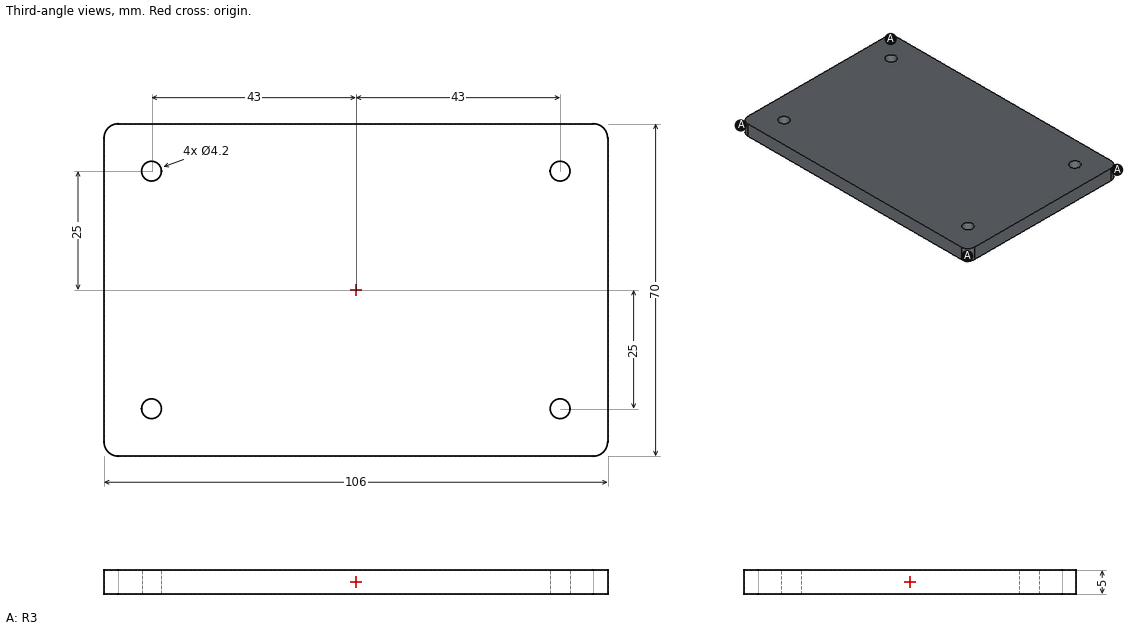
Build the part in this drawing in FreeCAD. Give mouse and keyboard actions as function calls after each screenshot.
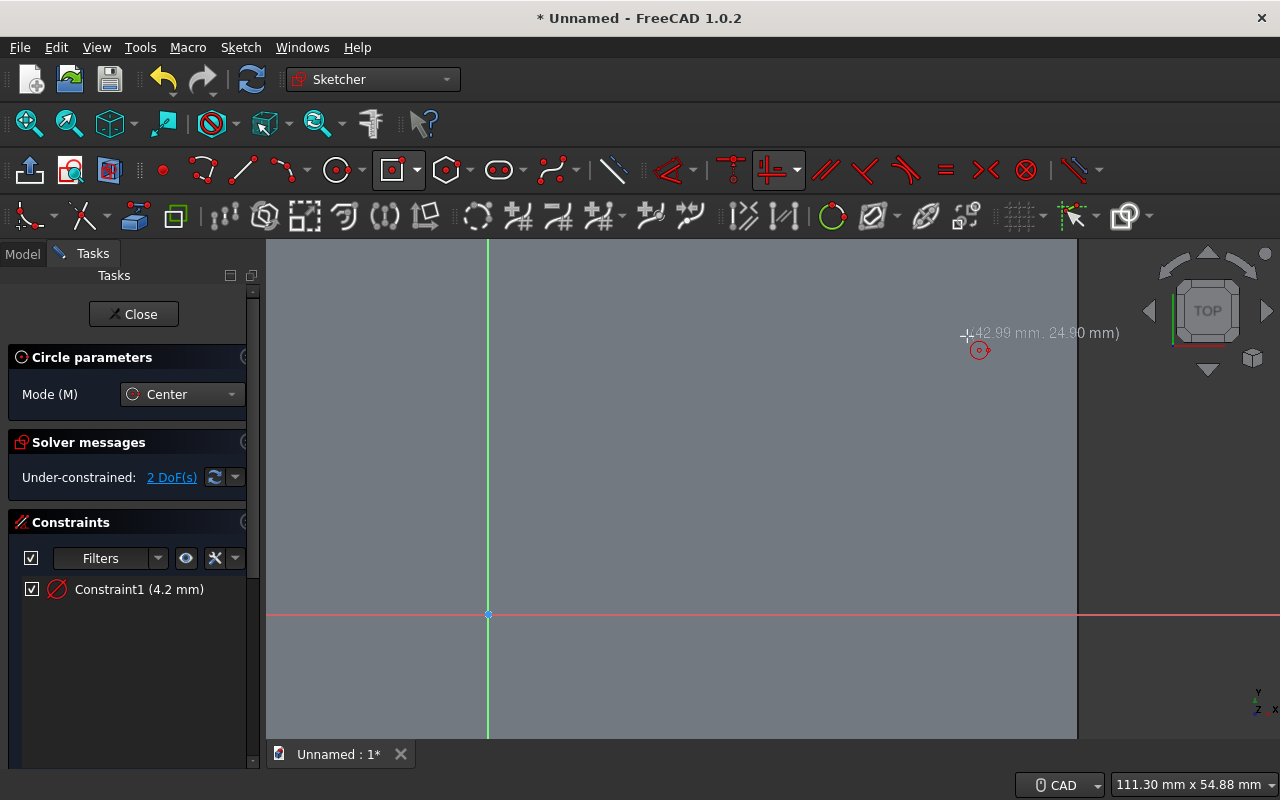
click(967, 337)
move(983, 320)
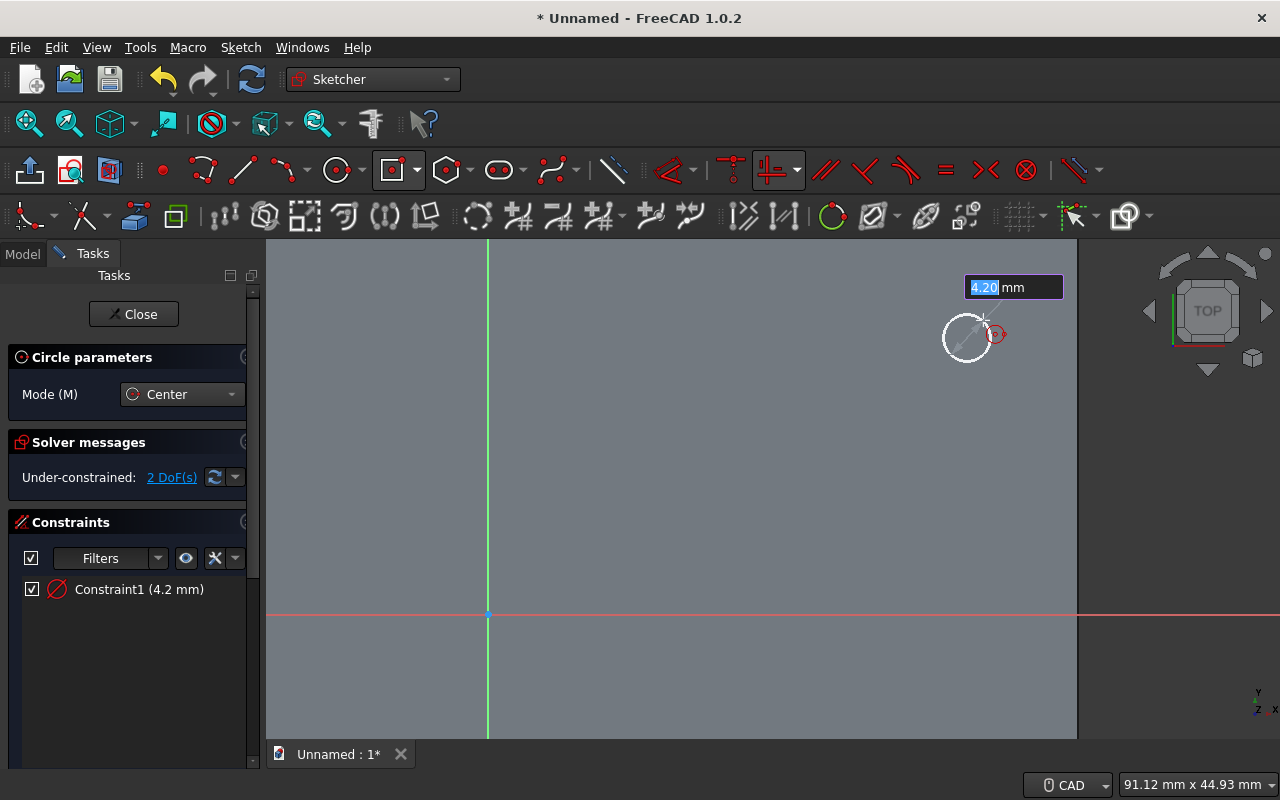
text(4.2)
key(Return)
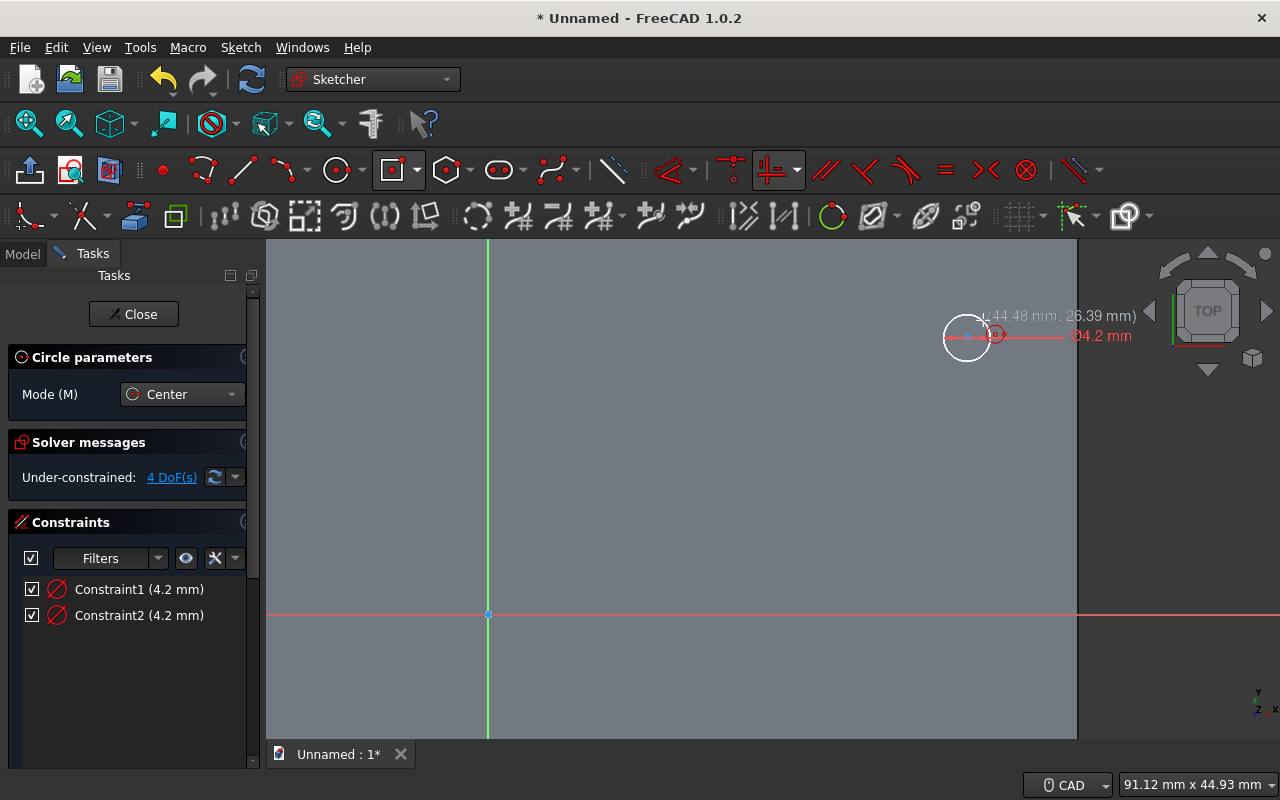
scroll(968, 336, down, 3)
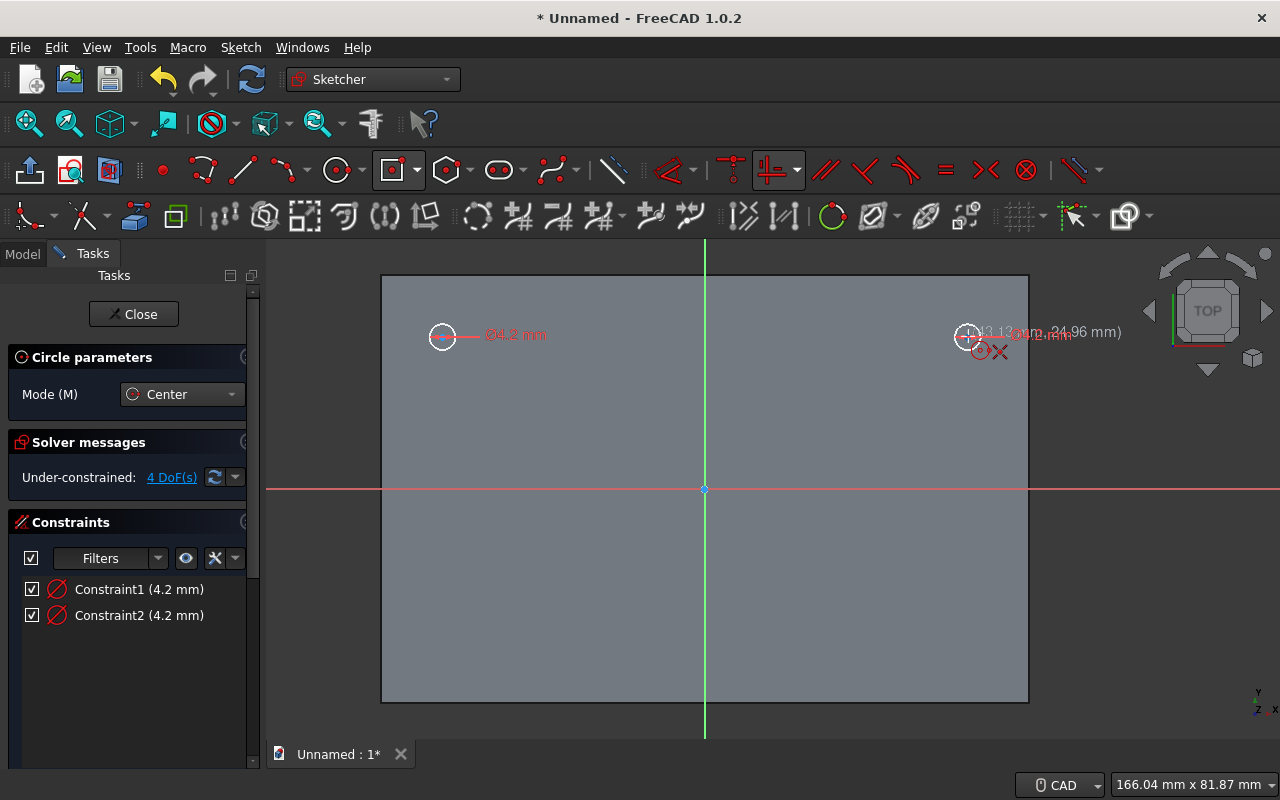
scroll(968, 642, up, 3)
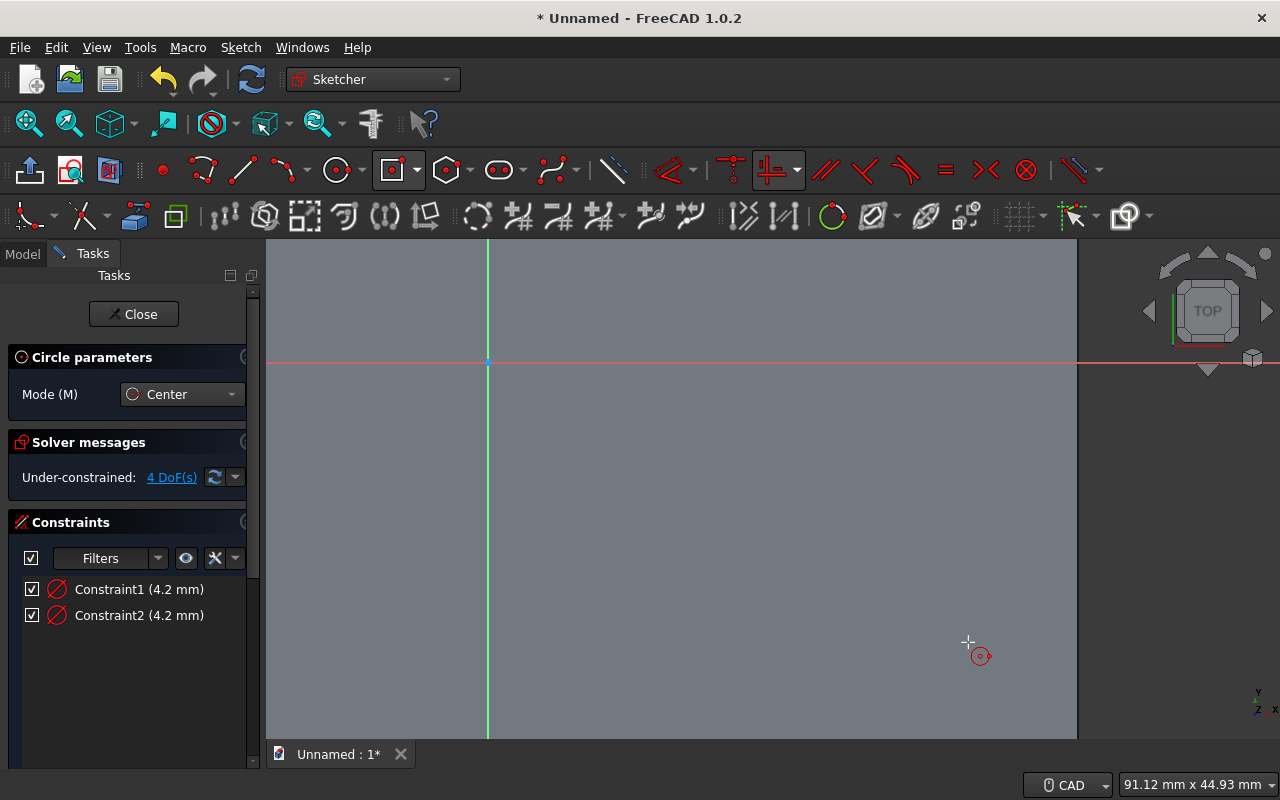
click(967, 641)
move(983, 624)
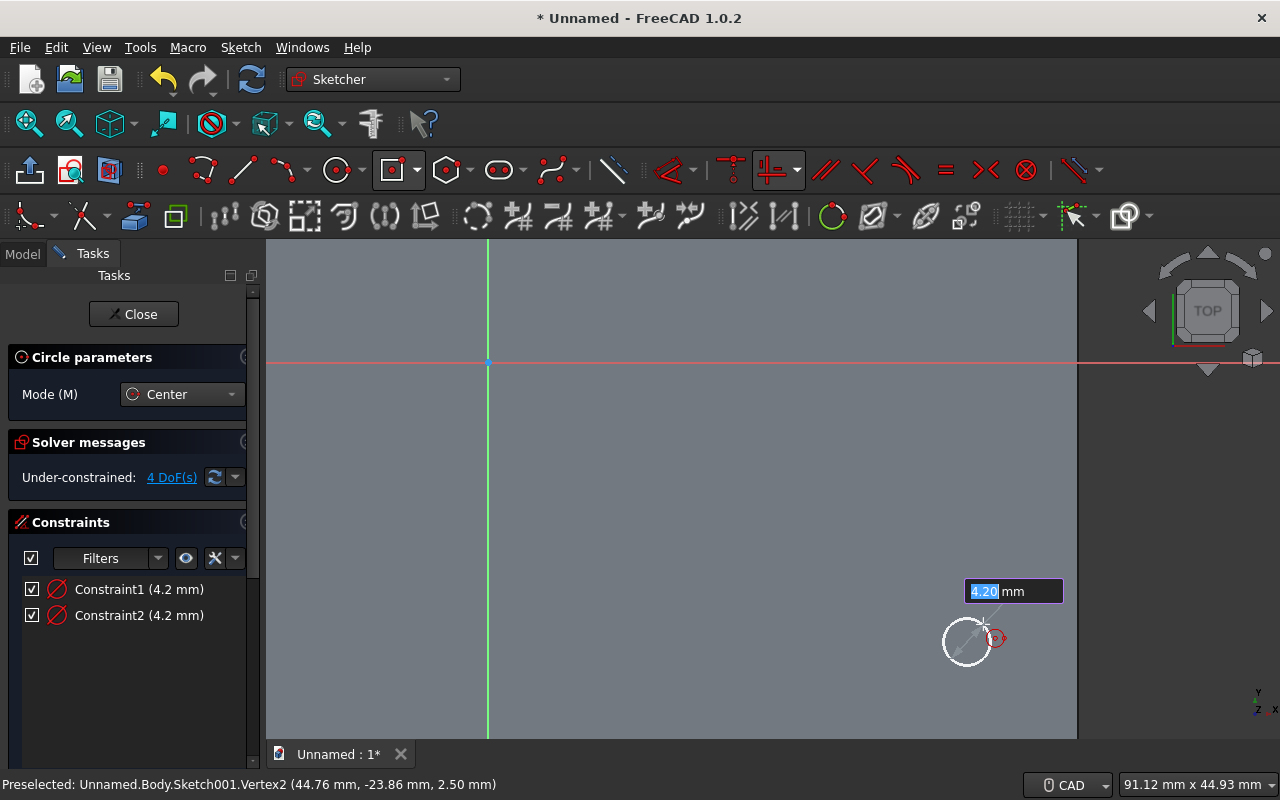
text(4.2)
key(Return)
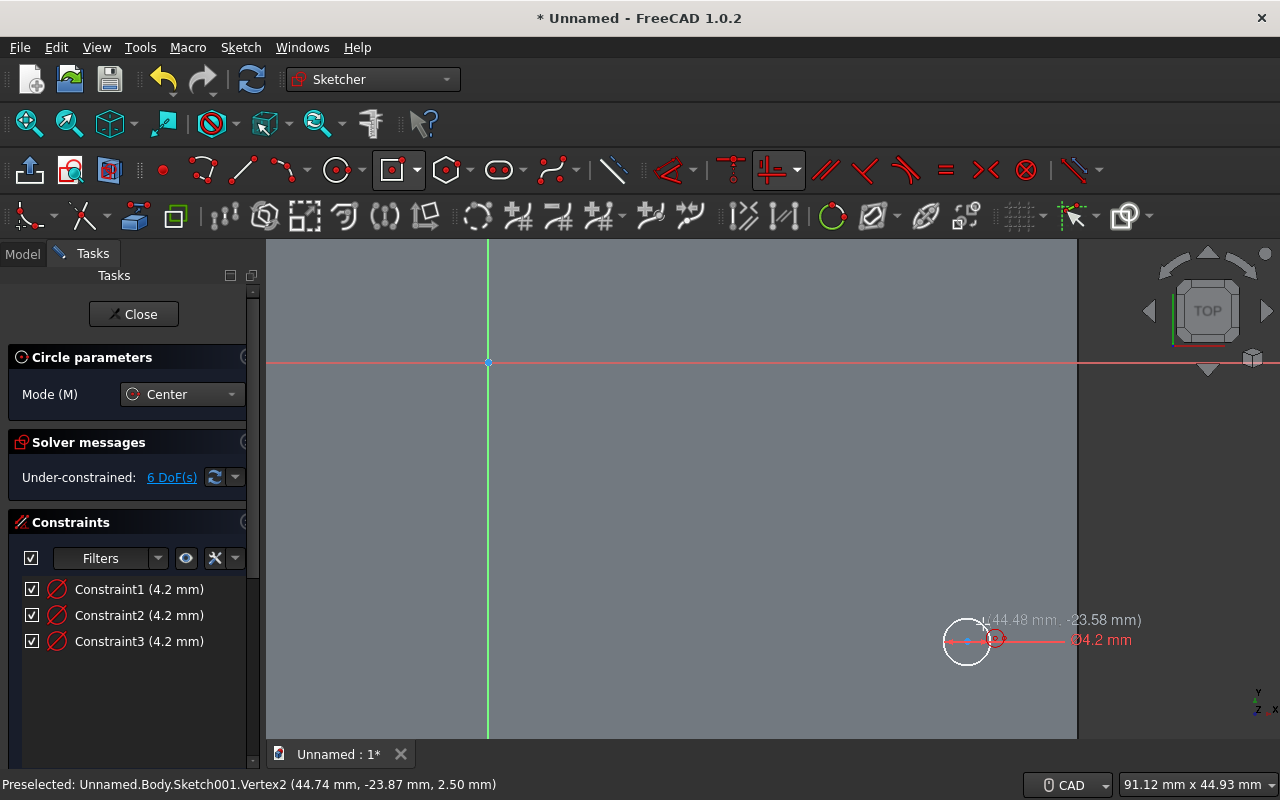
scroll(968, 643, down, 3)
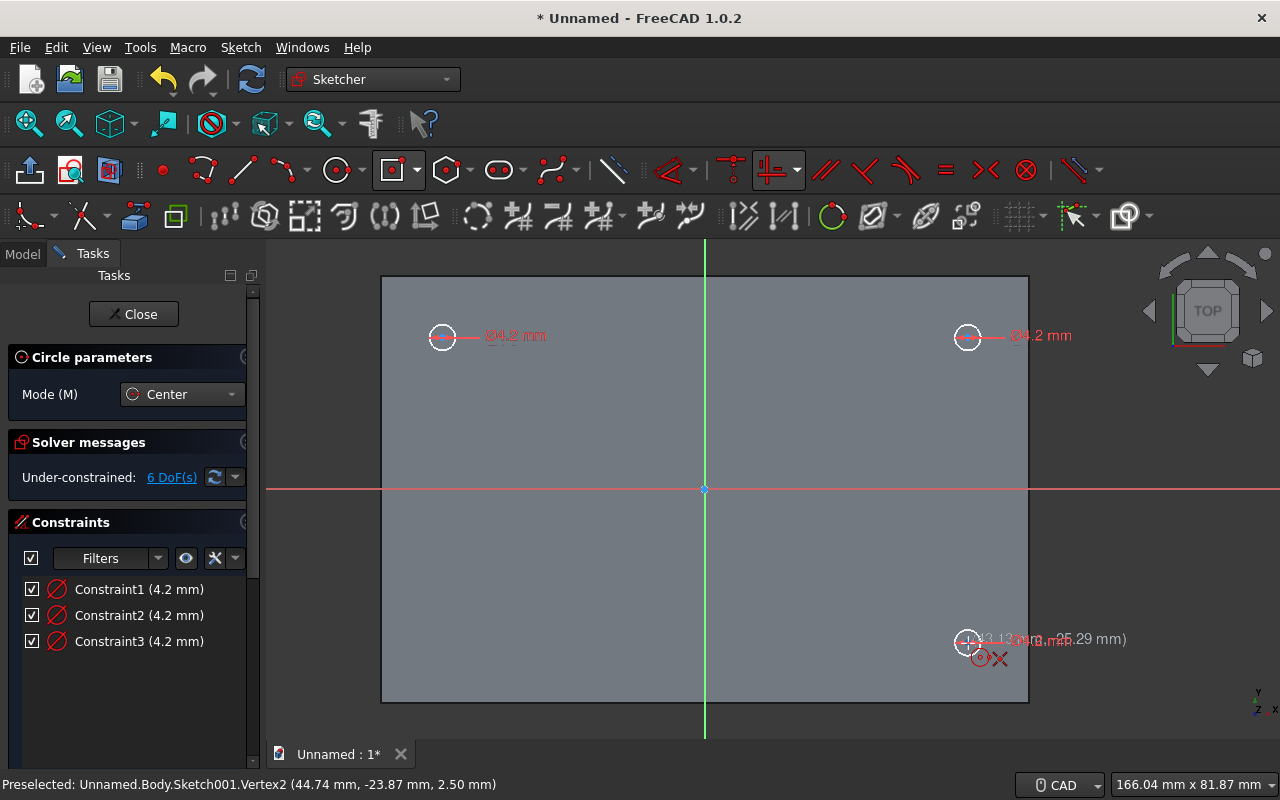
scroll(442, 642, up, 3)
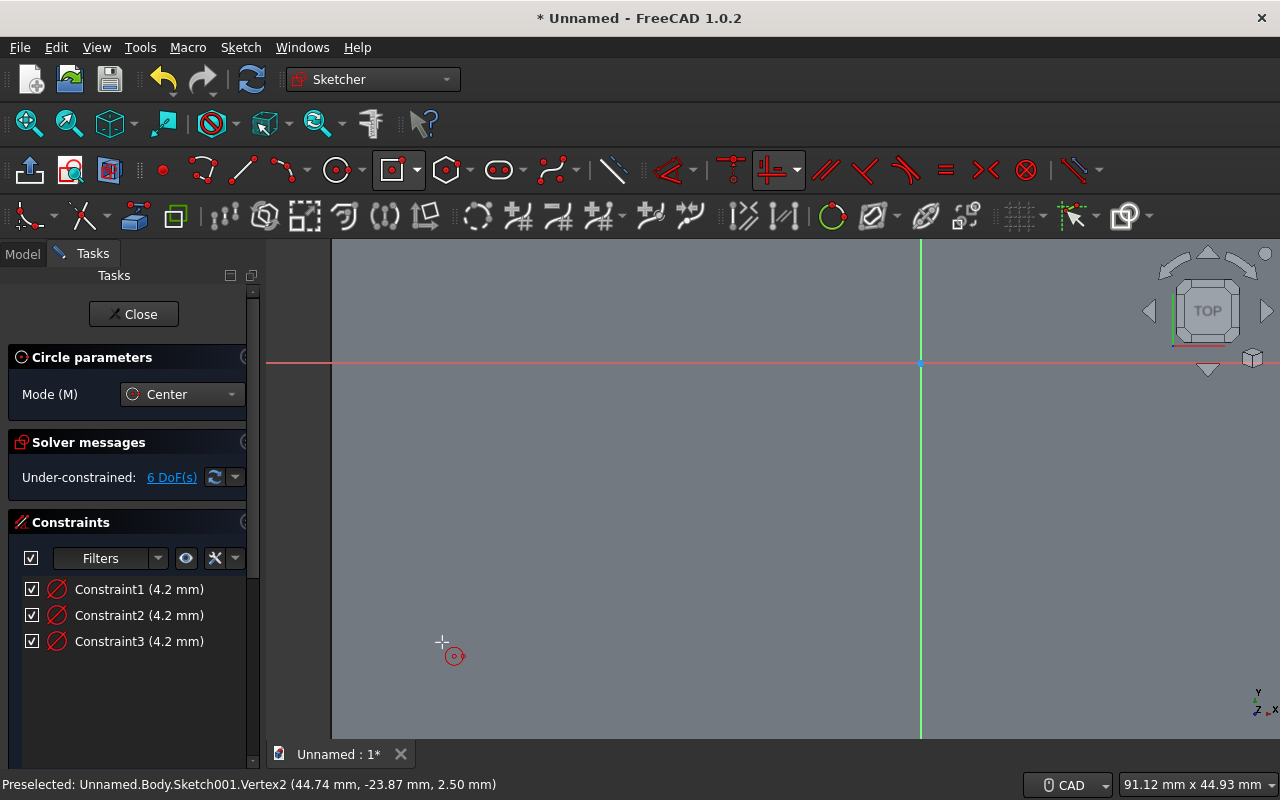
click(442, 642)
move(459, 625)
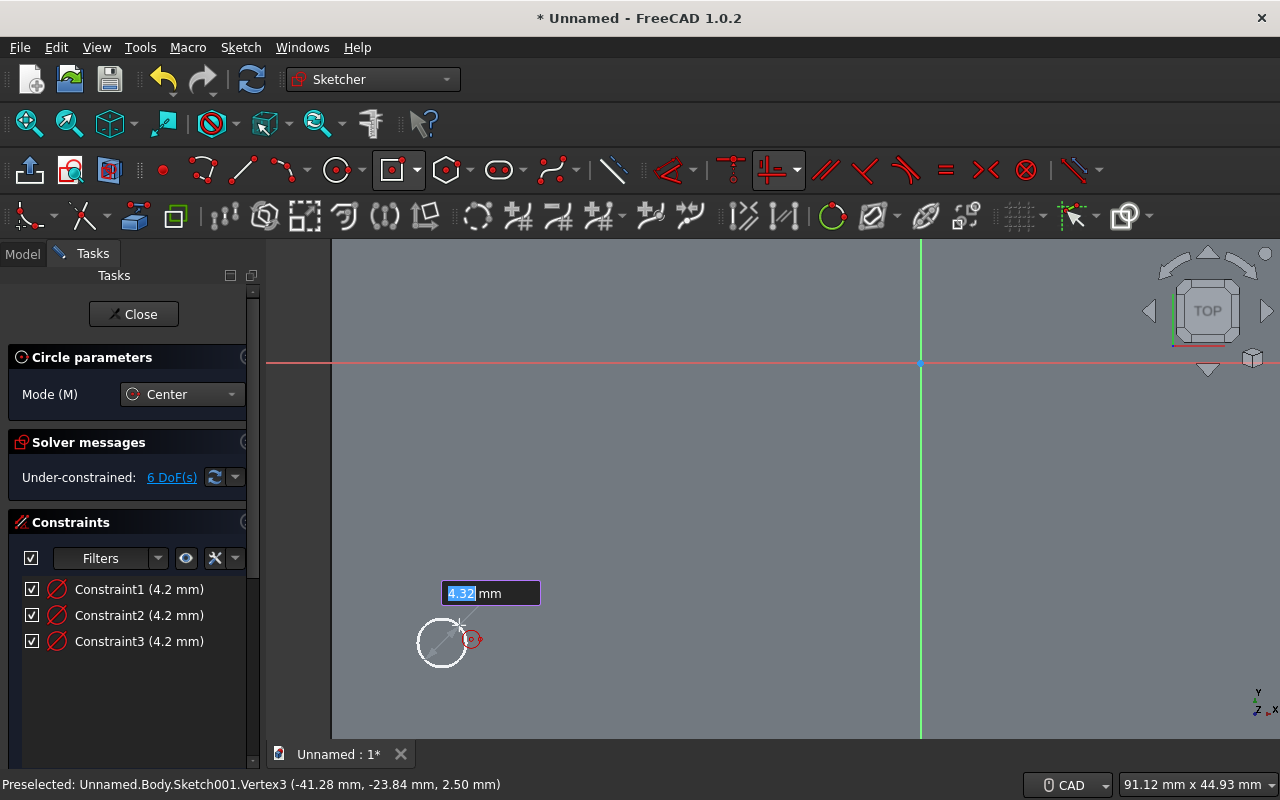
text(4.2)
key(Return)
key(Escape)